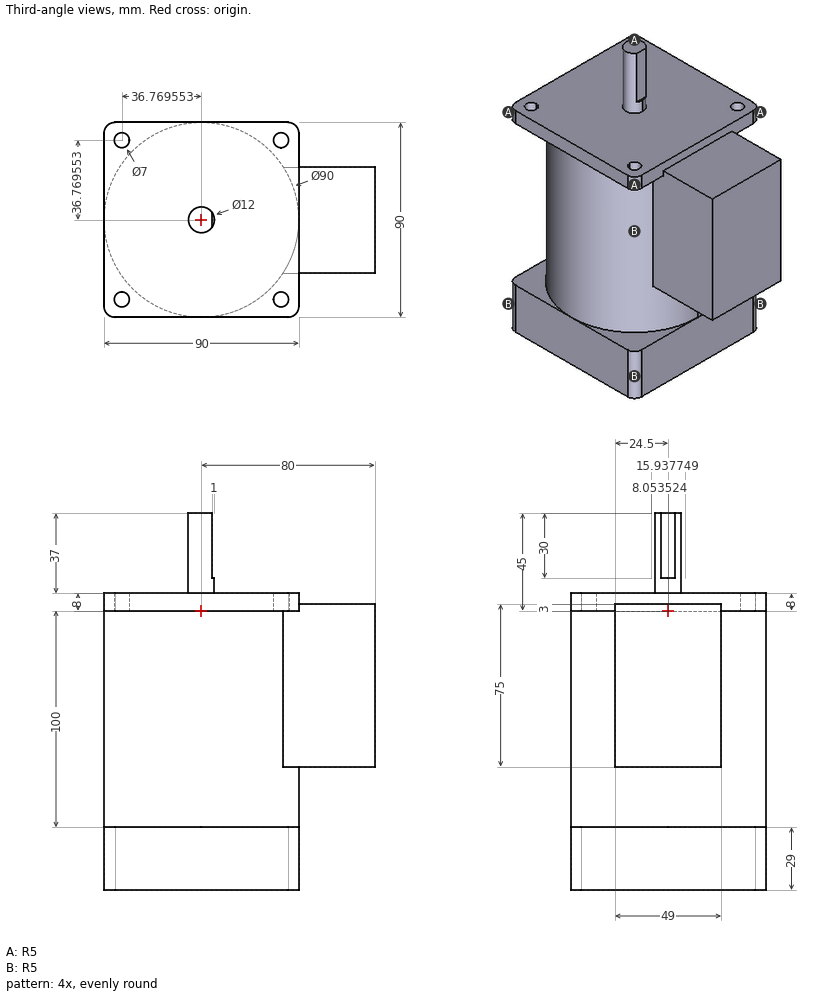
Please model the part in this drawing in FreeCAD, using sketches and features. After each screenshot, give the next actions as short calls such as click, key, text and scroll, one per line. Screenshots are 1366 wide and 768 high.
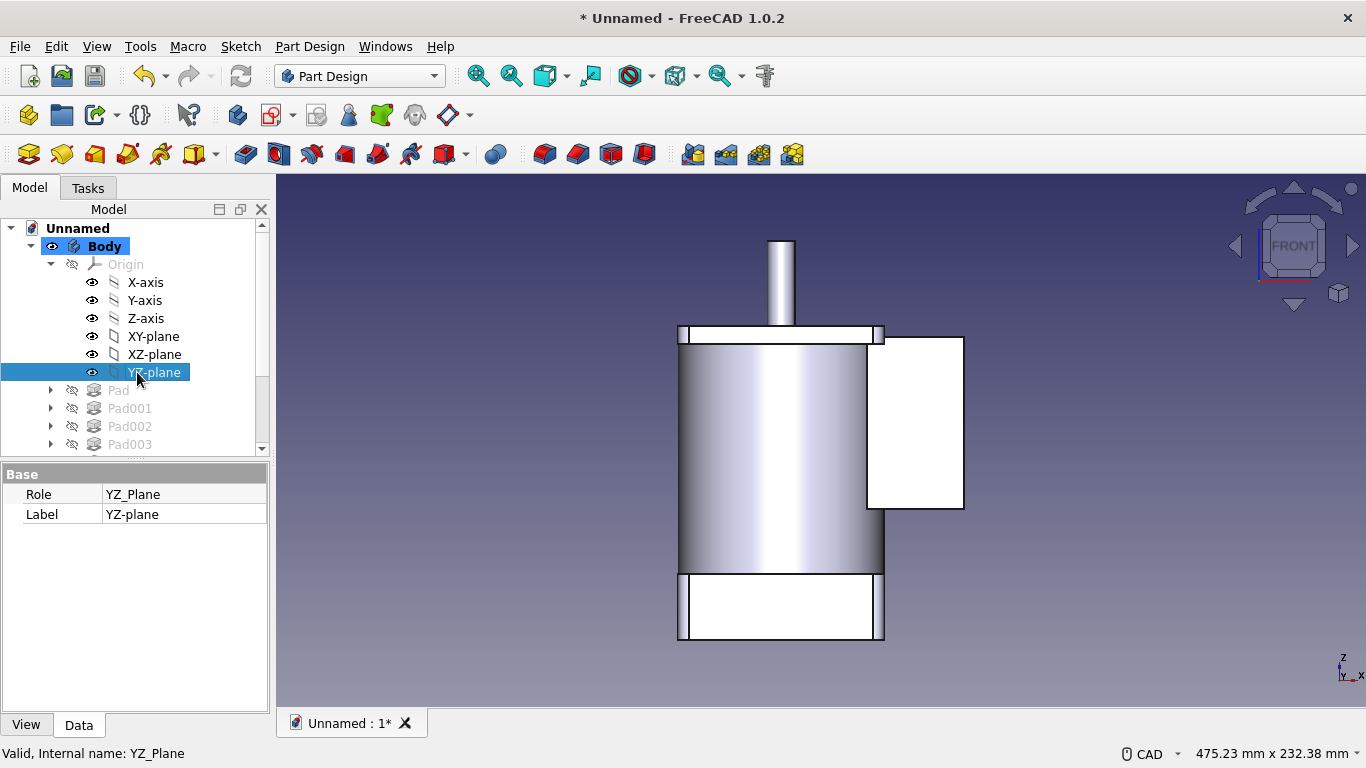
click(448, 116)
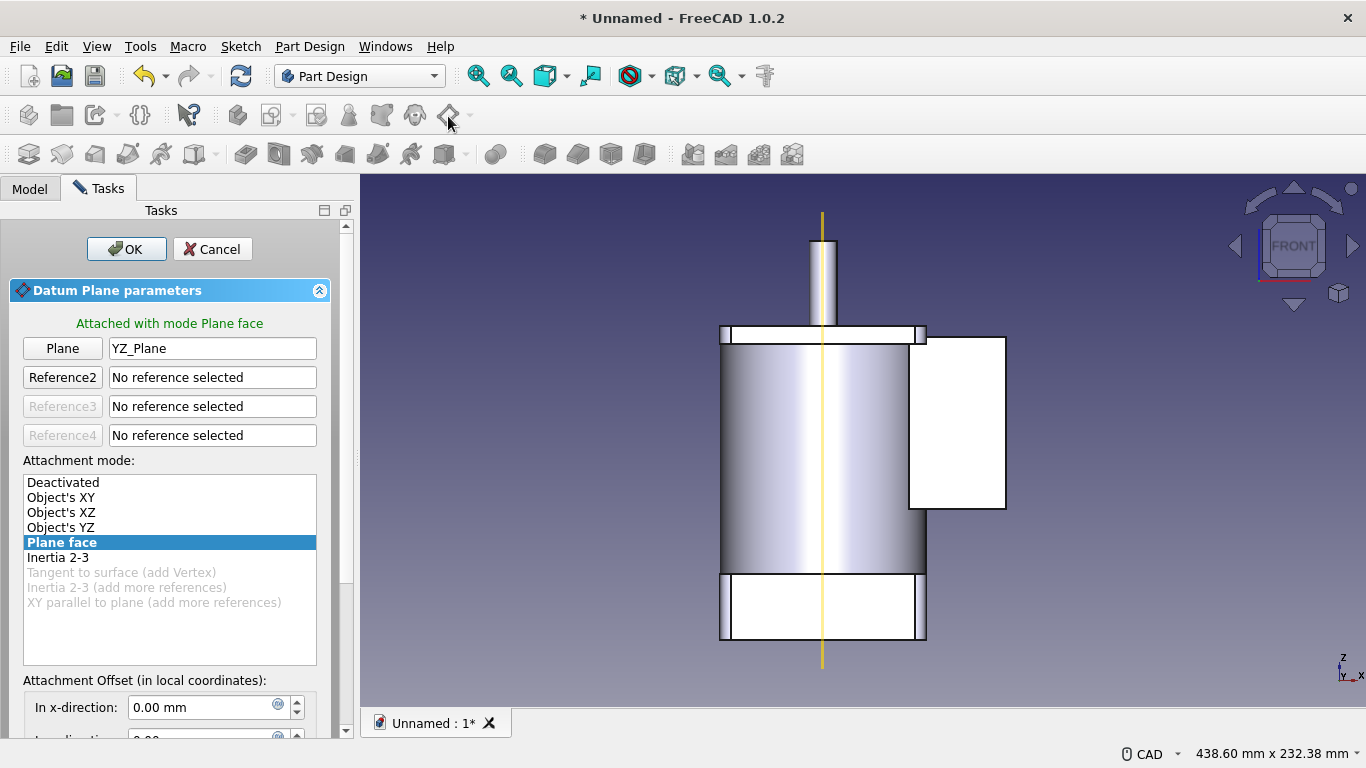
scroll(346, 479, down, 2)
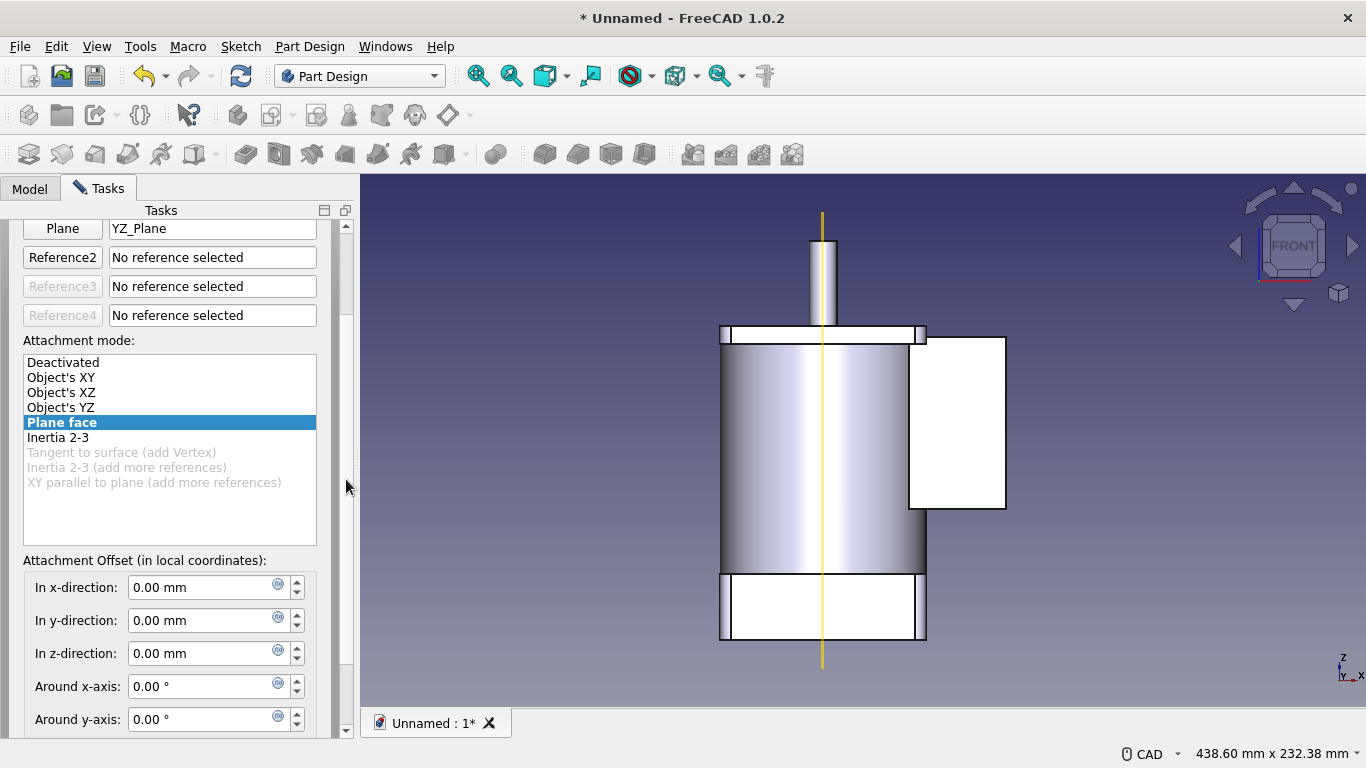
triple_click(210, 654)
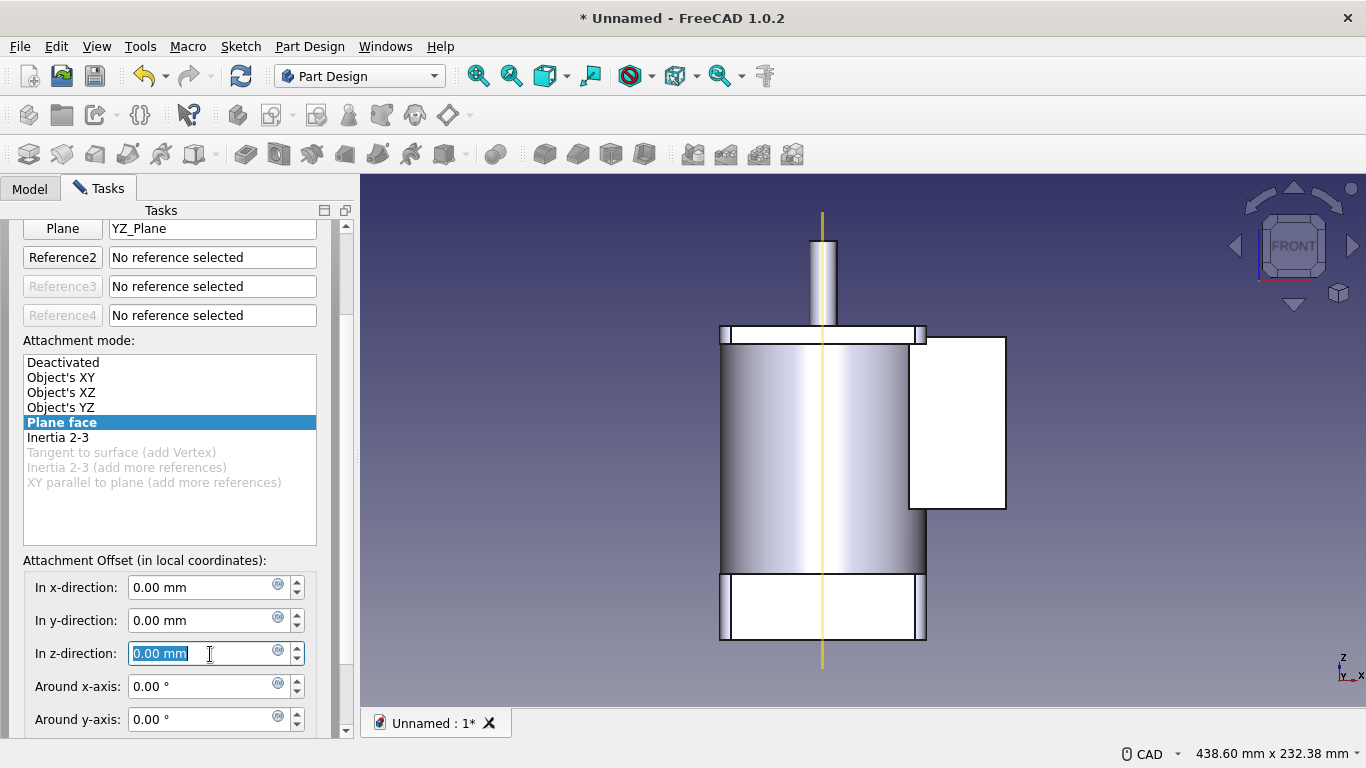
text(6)
key(Tab)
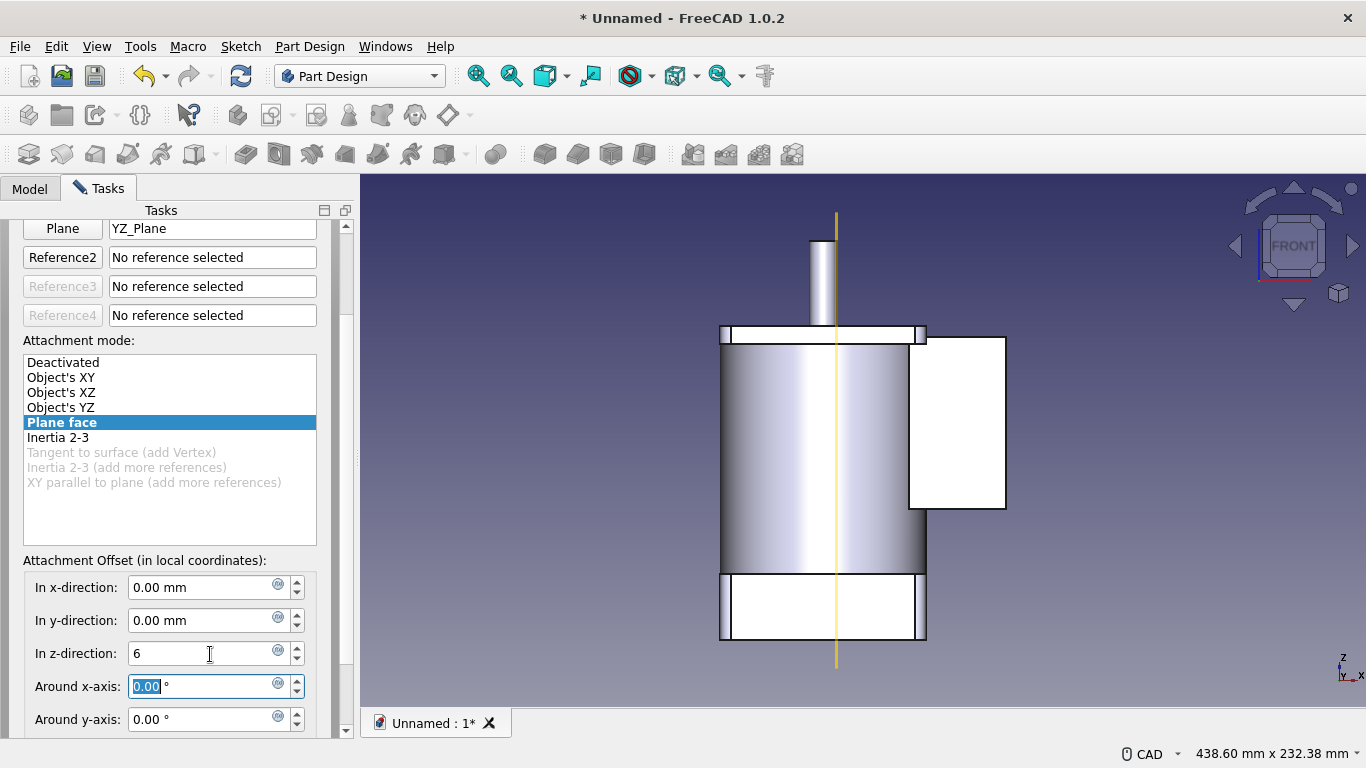
scroll(346, 479, up, 3)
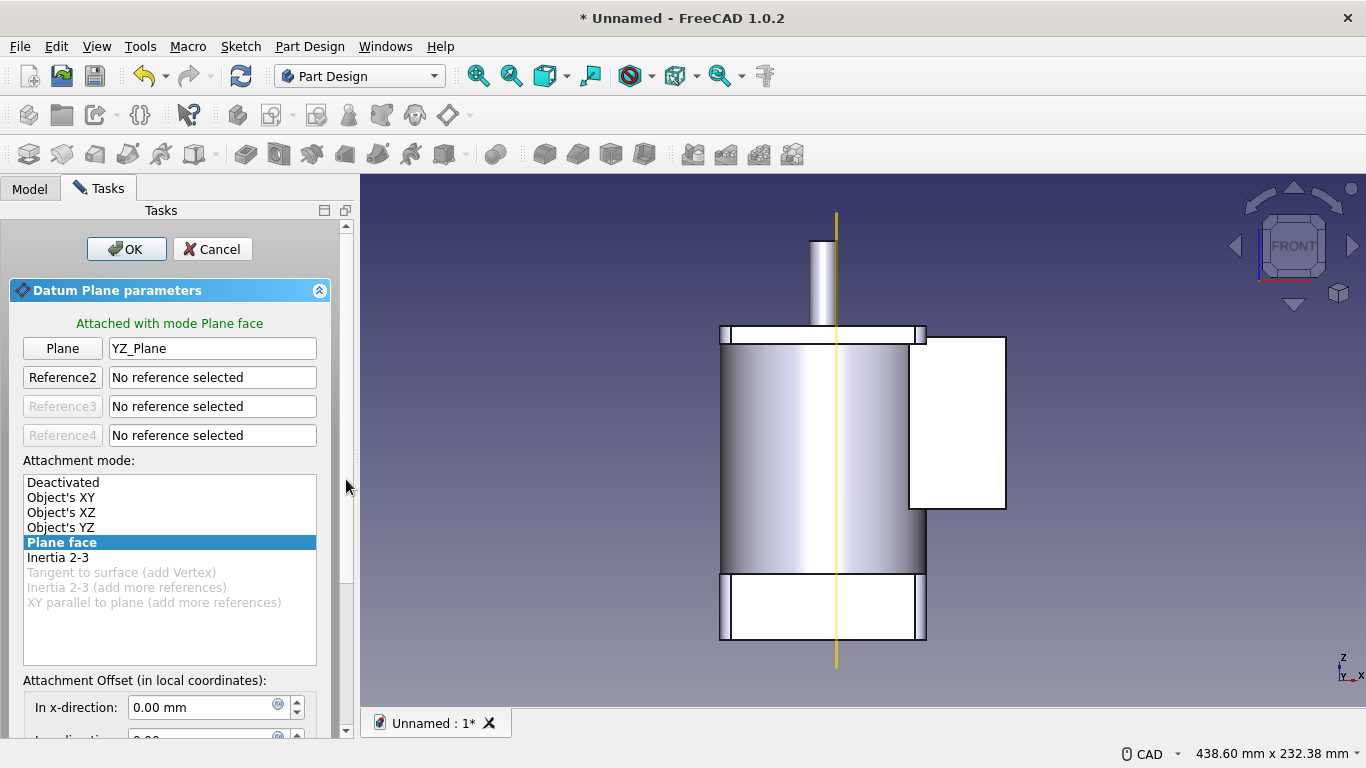
click(127, 249)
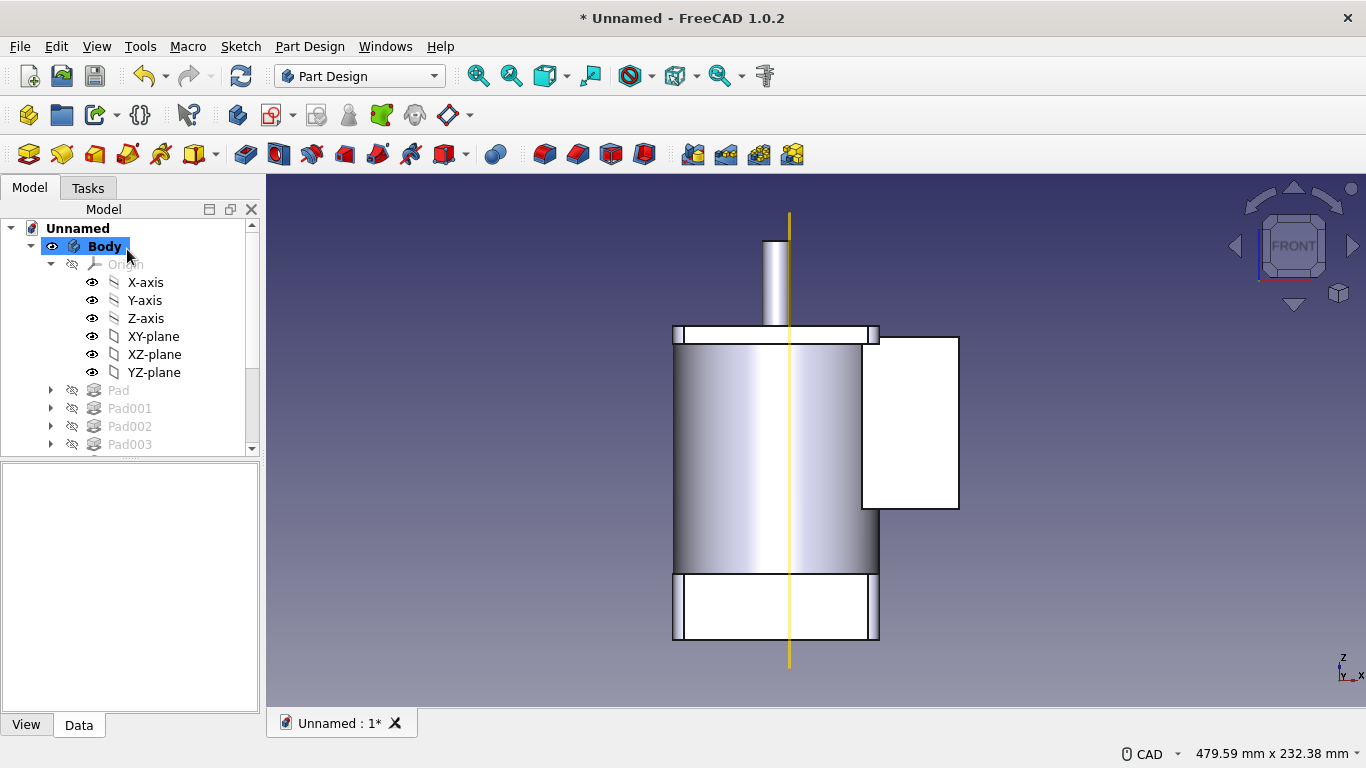
scroll(101, 332, down, 3)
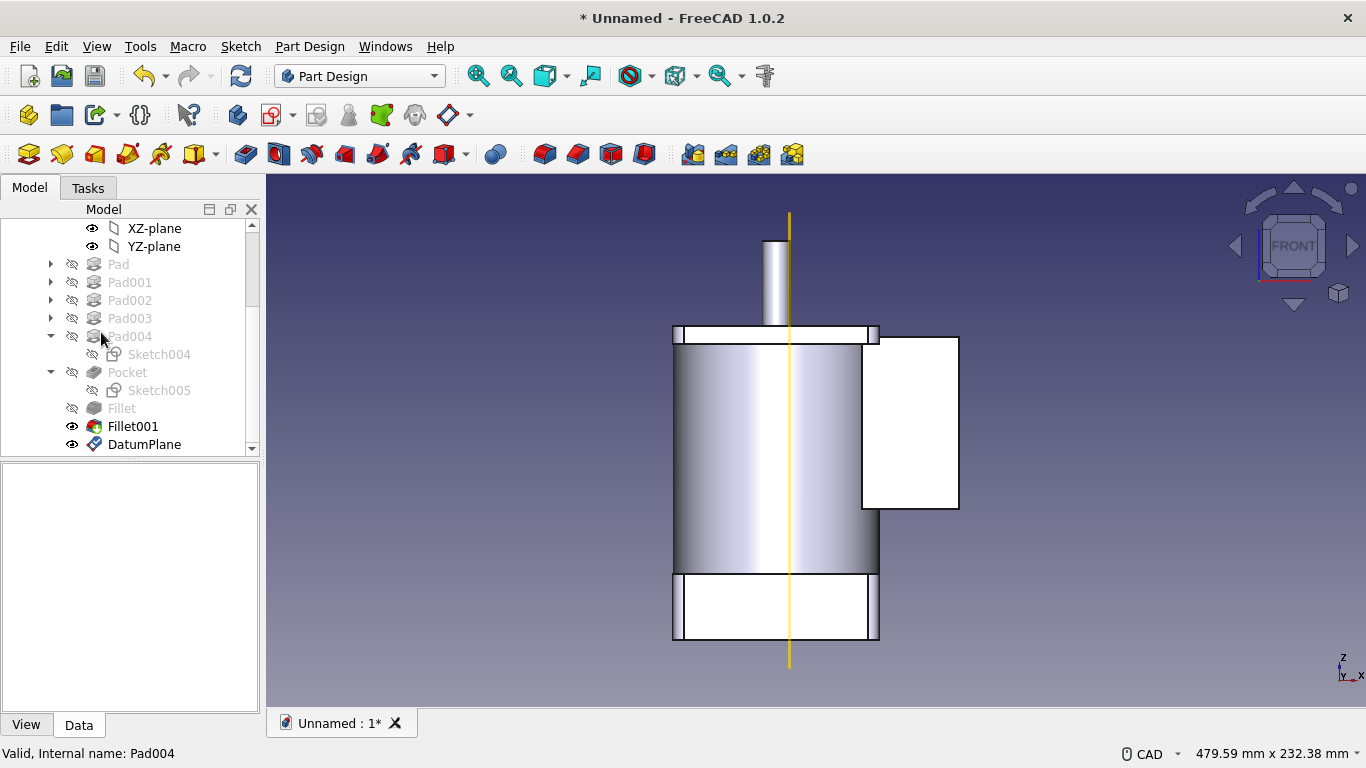
click(117, 444)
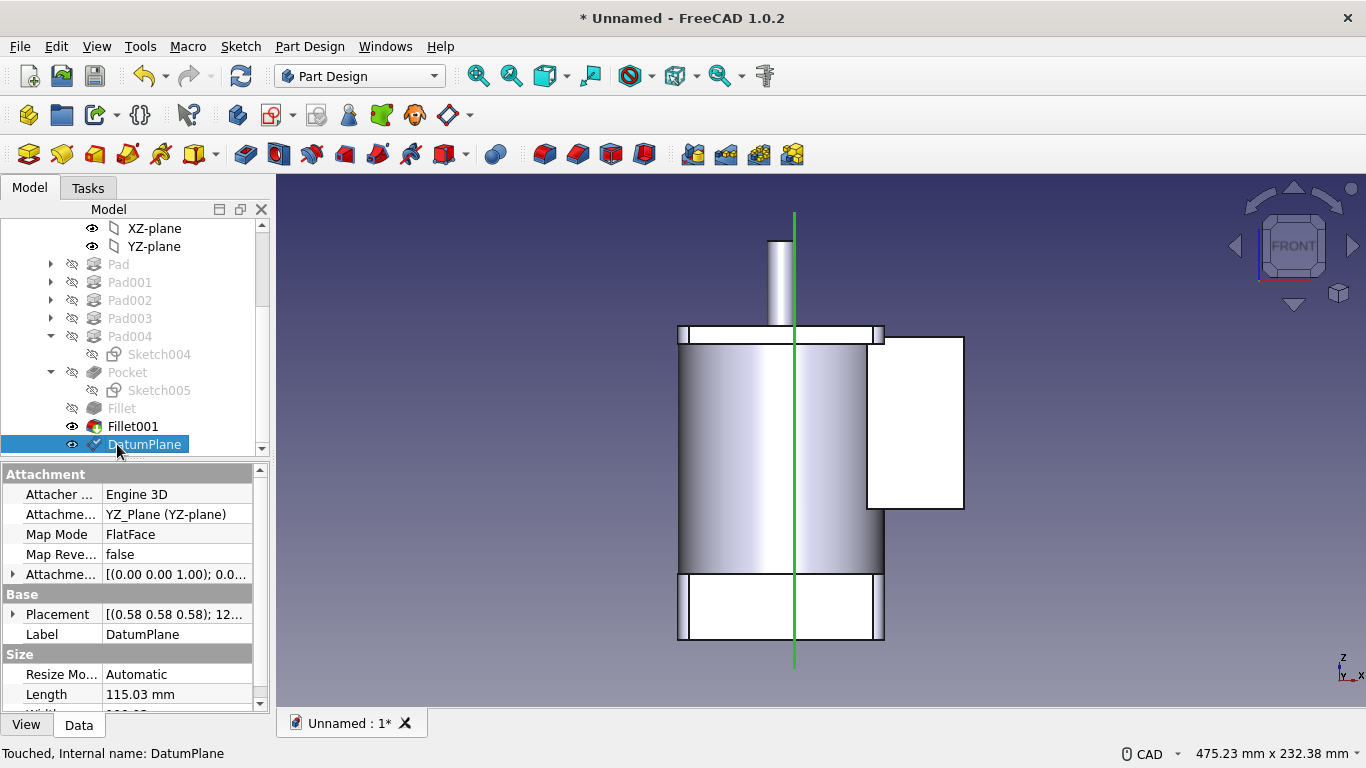
click(270, 116)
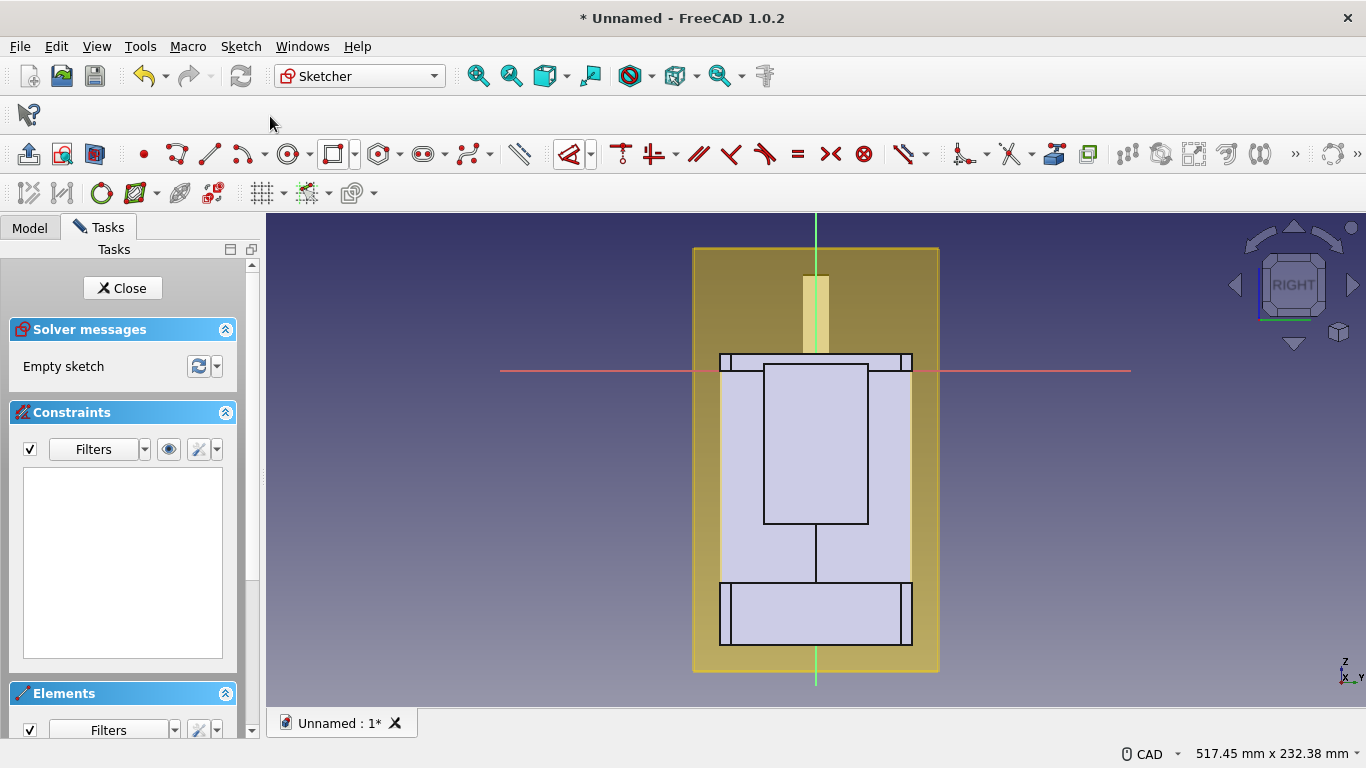
click(95, 154)